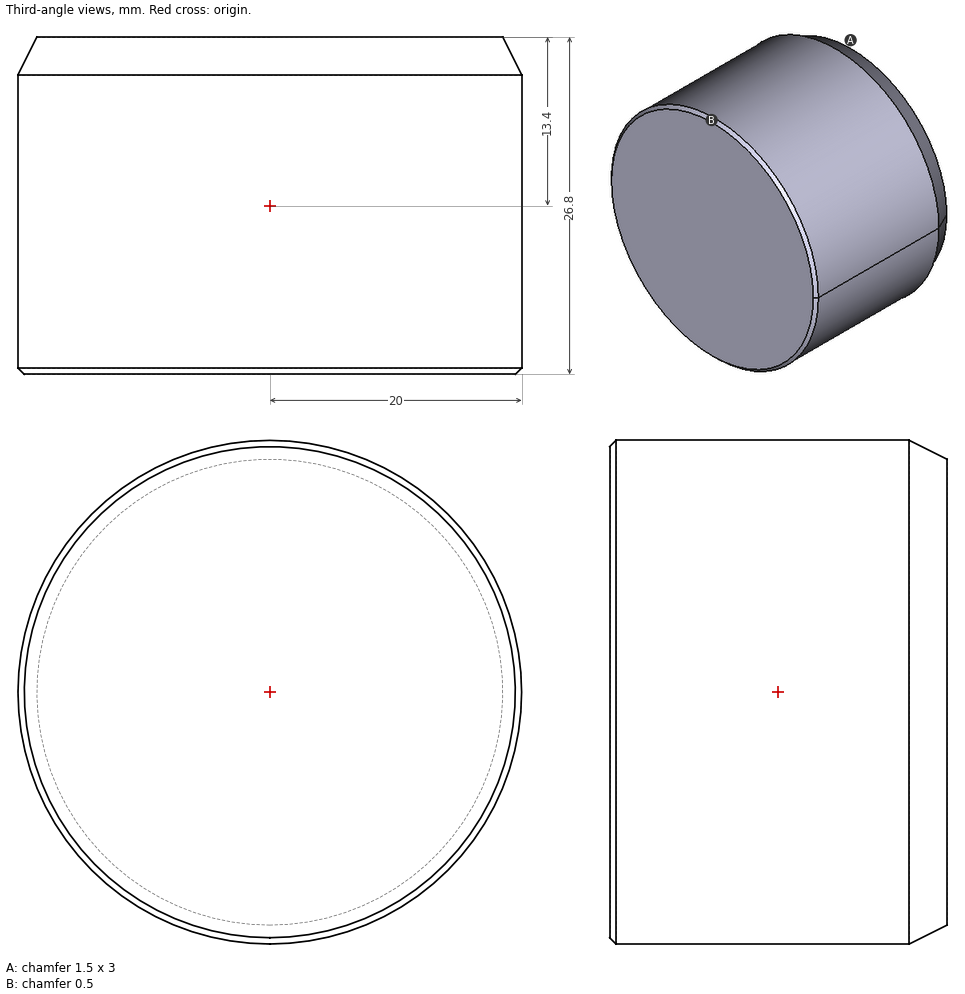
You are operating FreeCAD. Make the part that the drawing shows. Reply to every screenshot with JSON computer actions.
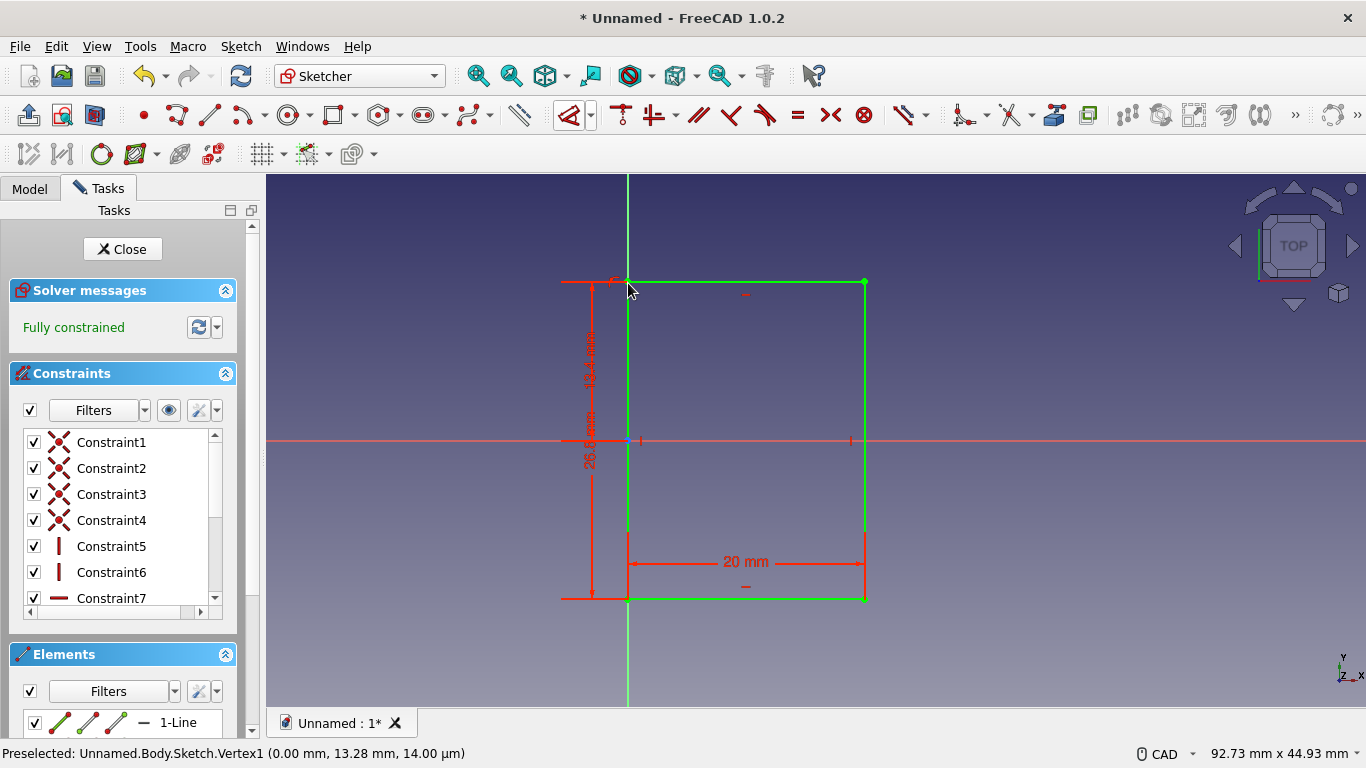
{"action": "left_click", "coordinate": [123, 249]}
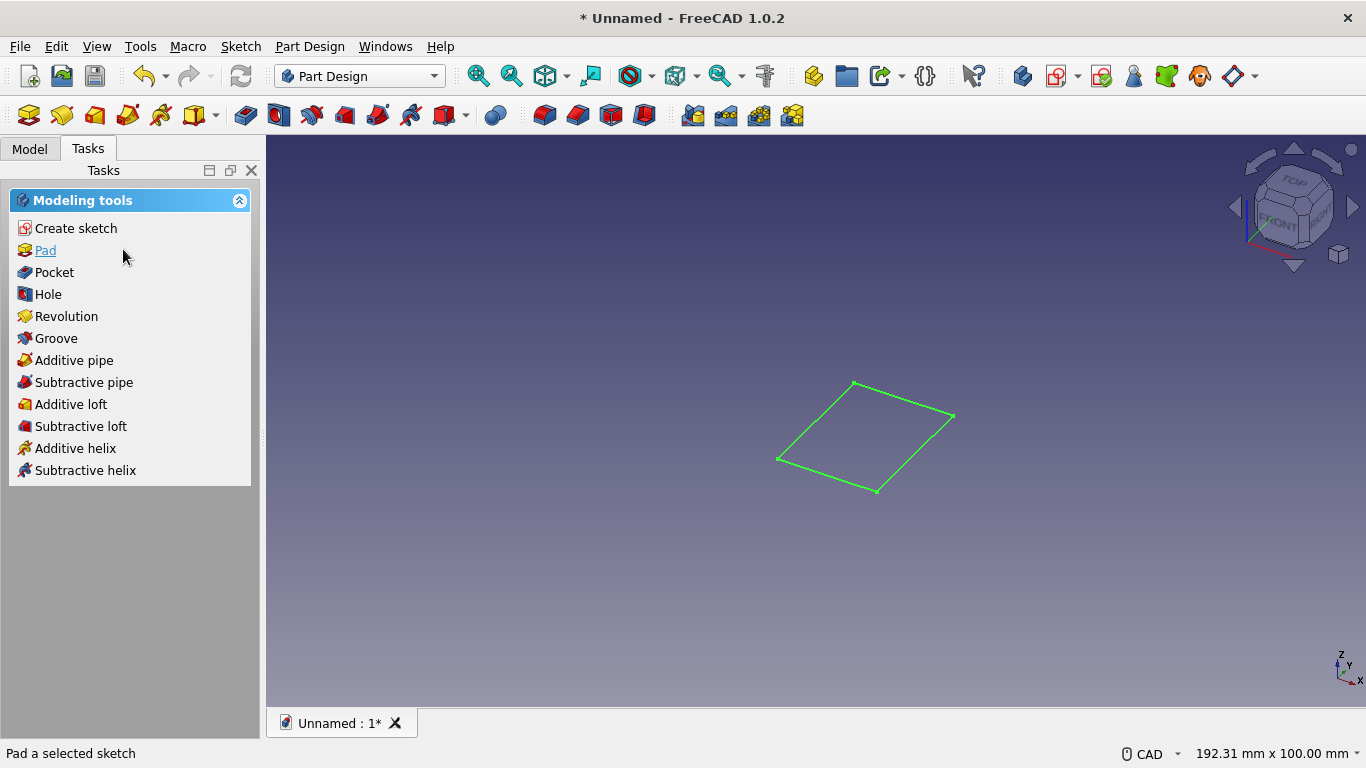
{"action": "left_click", "coordinate": [62, 116]}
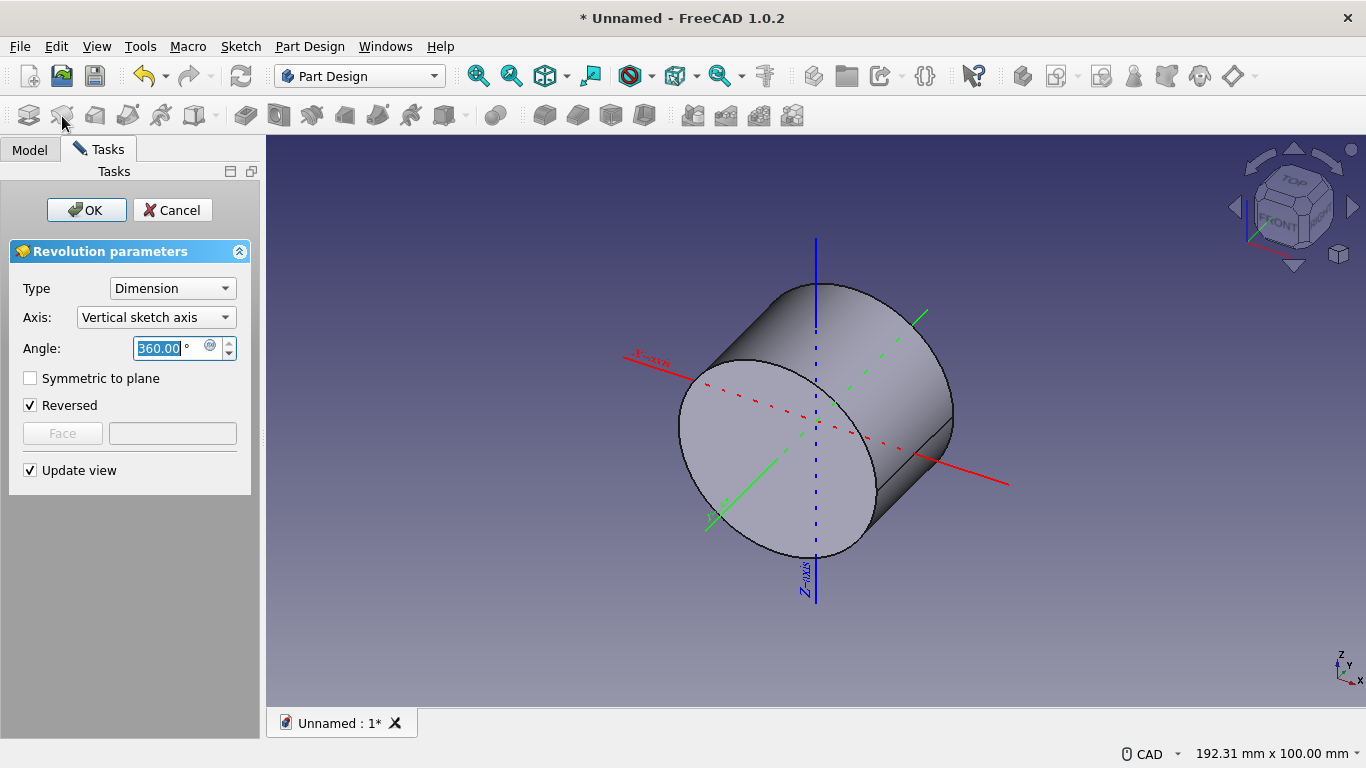
{"action": "left_click", "coordinate": [87, 210]}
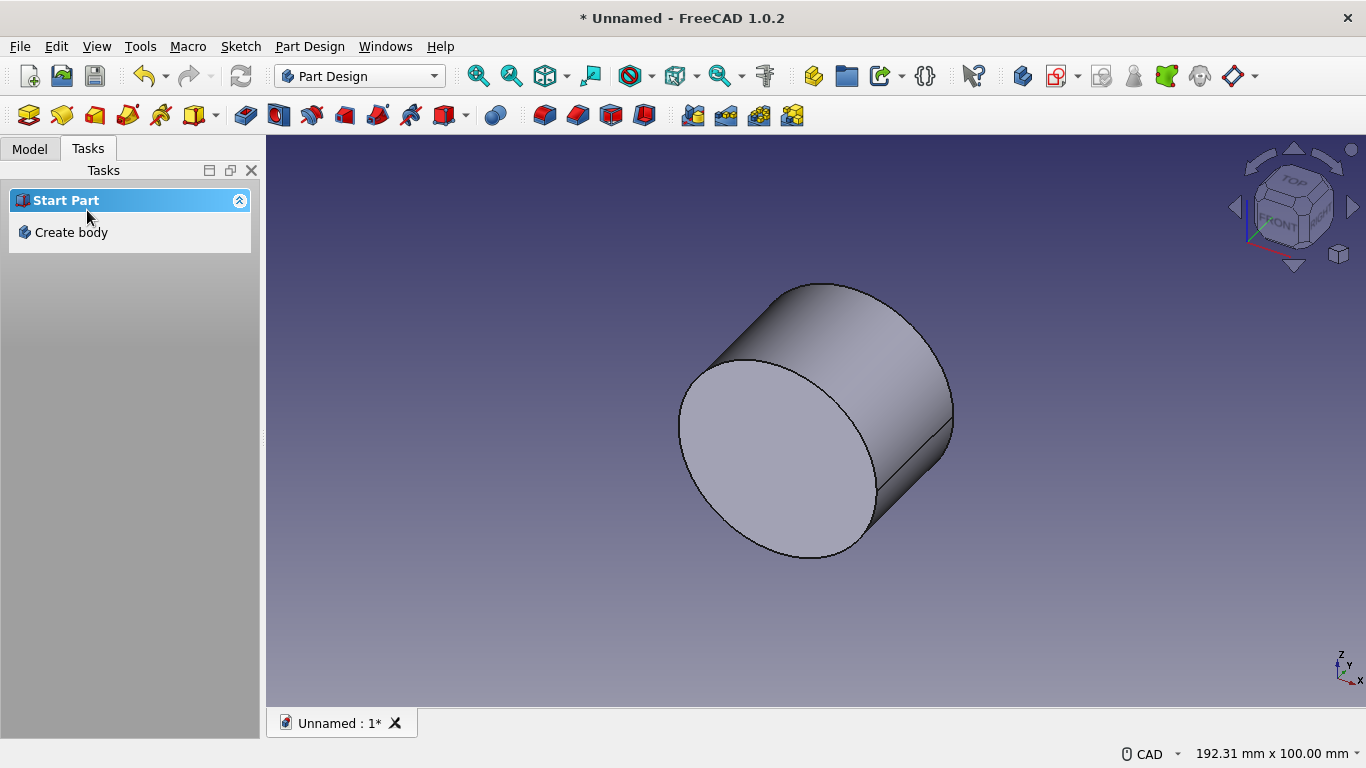
{"action": "key", "text": "0"}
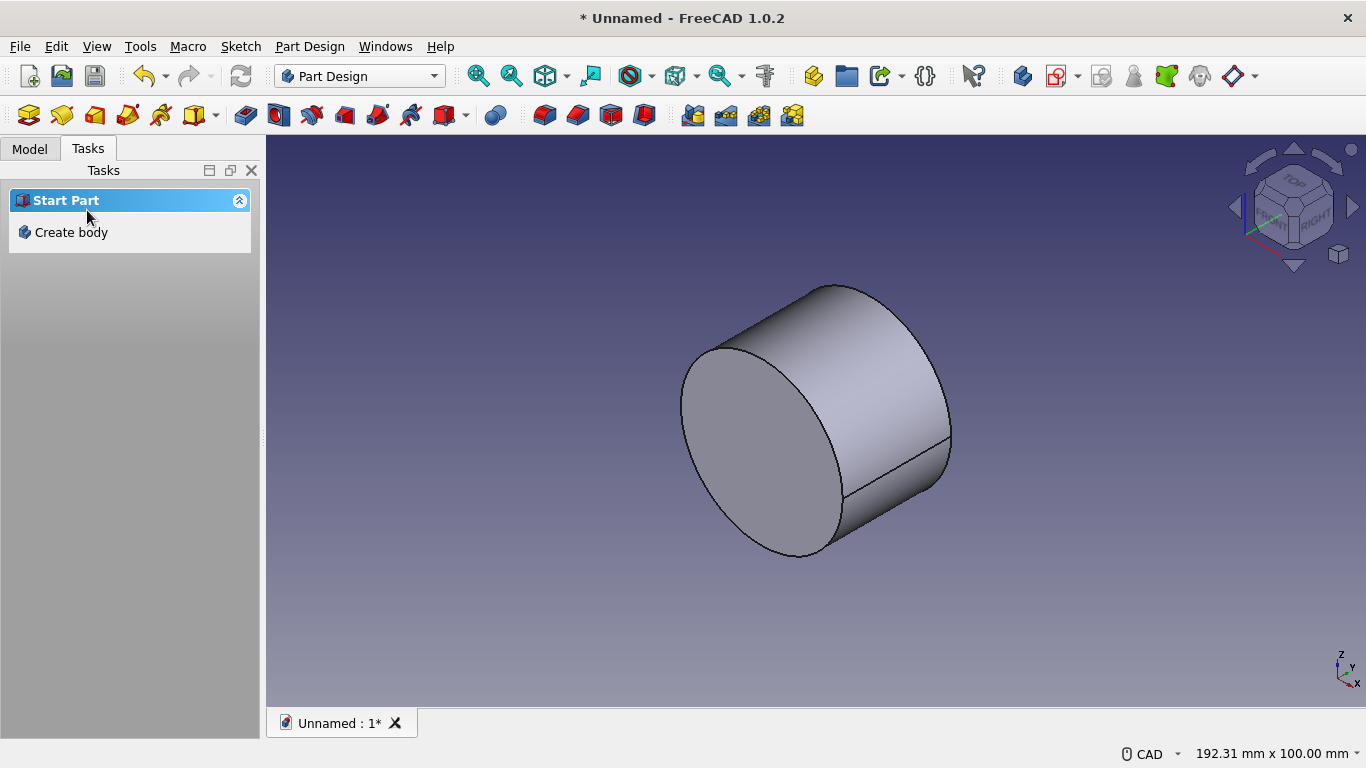
{"action": "key", "text": "2"}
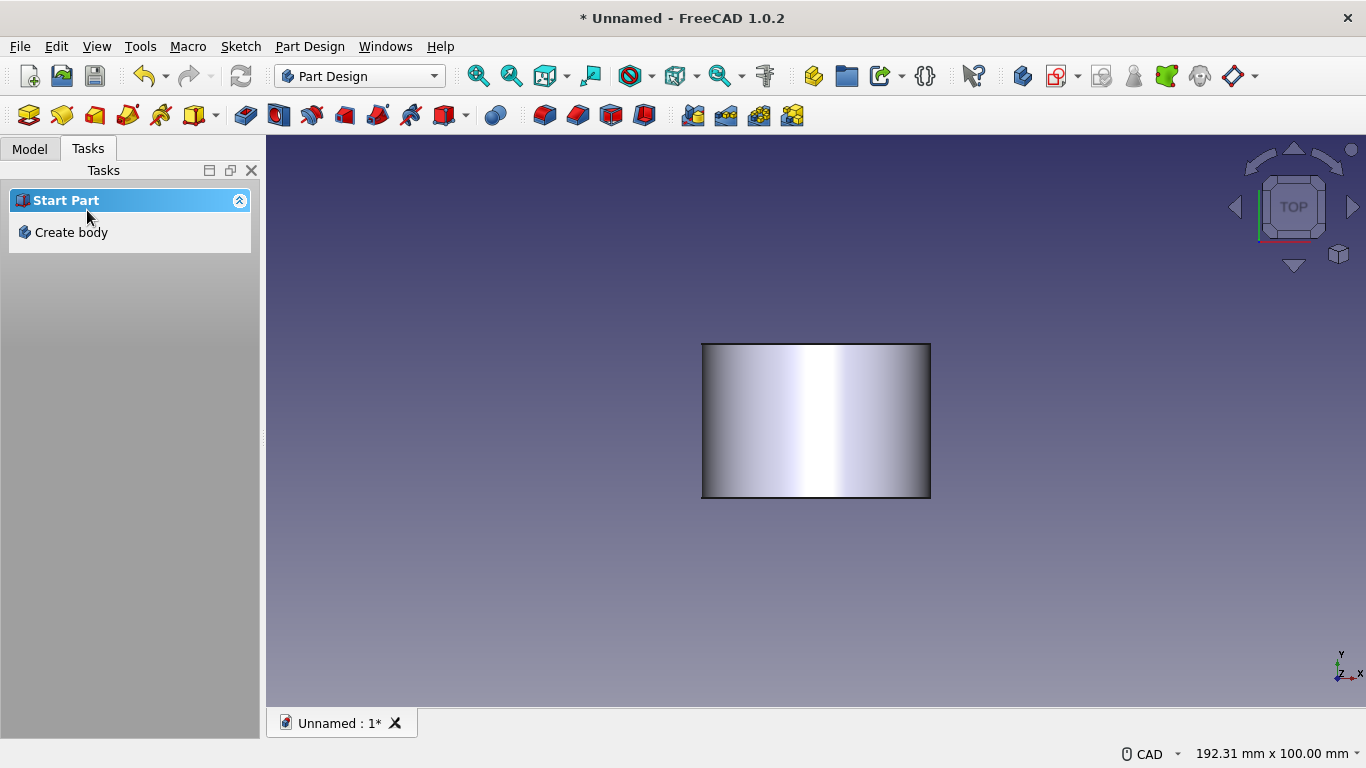
{"action": "key", "text": "v f"}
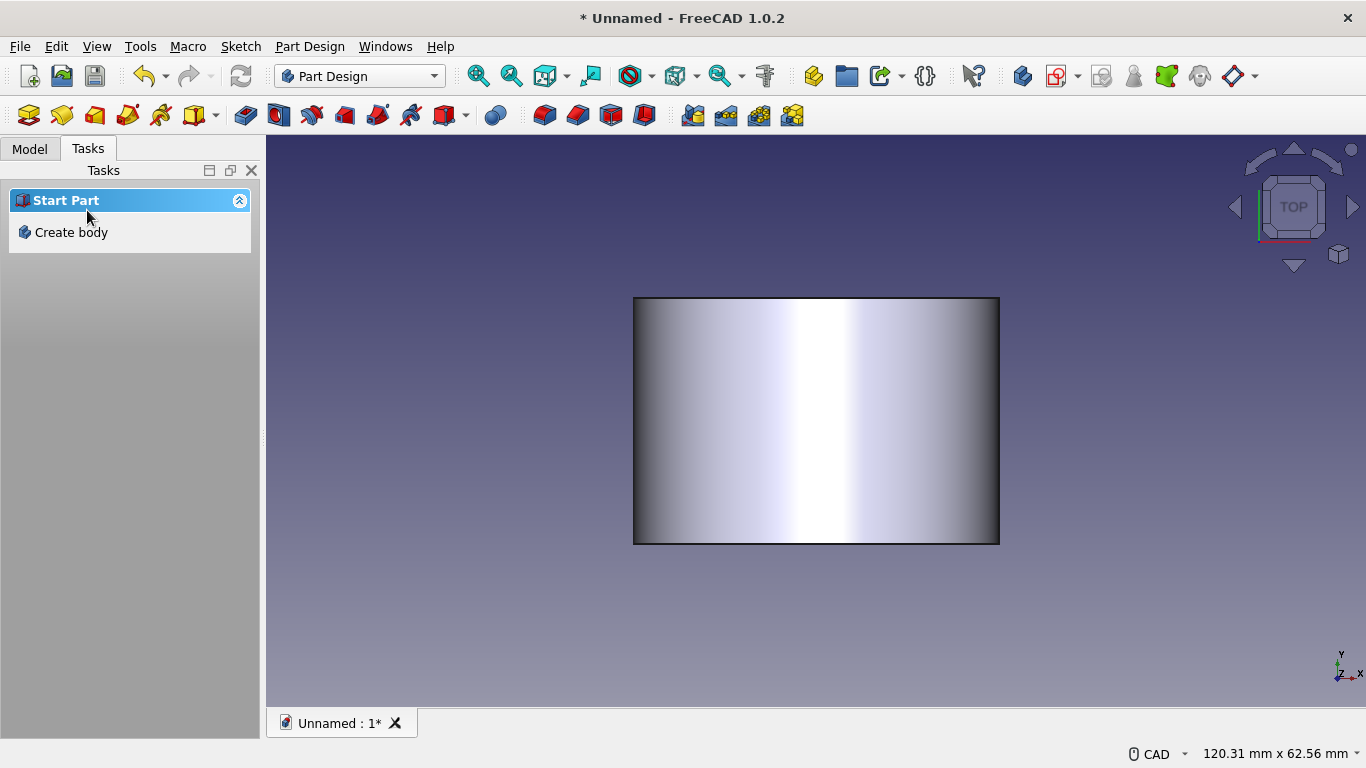
{"action": "left_click", "coordinate": [668, 297]}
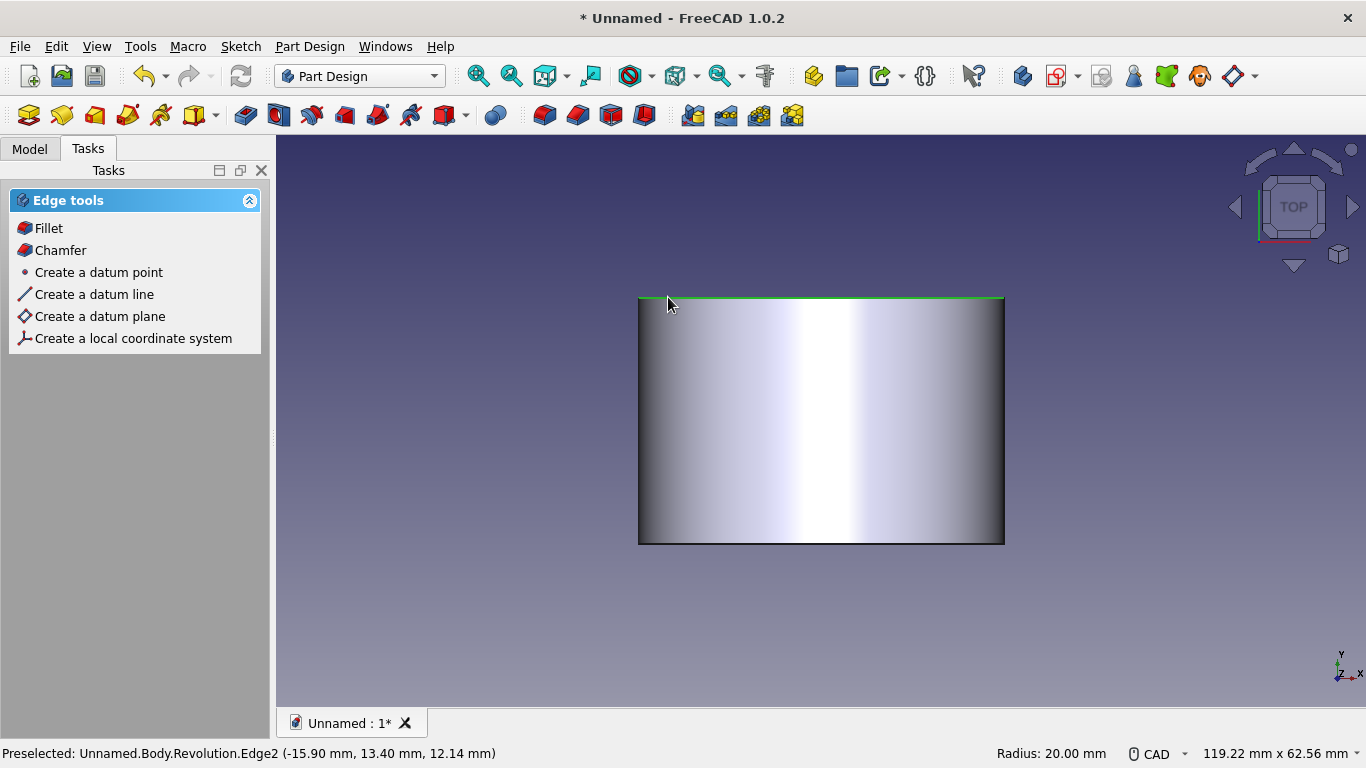
{"action": "left_click", "coordinate": [578, 116]}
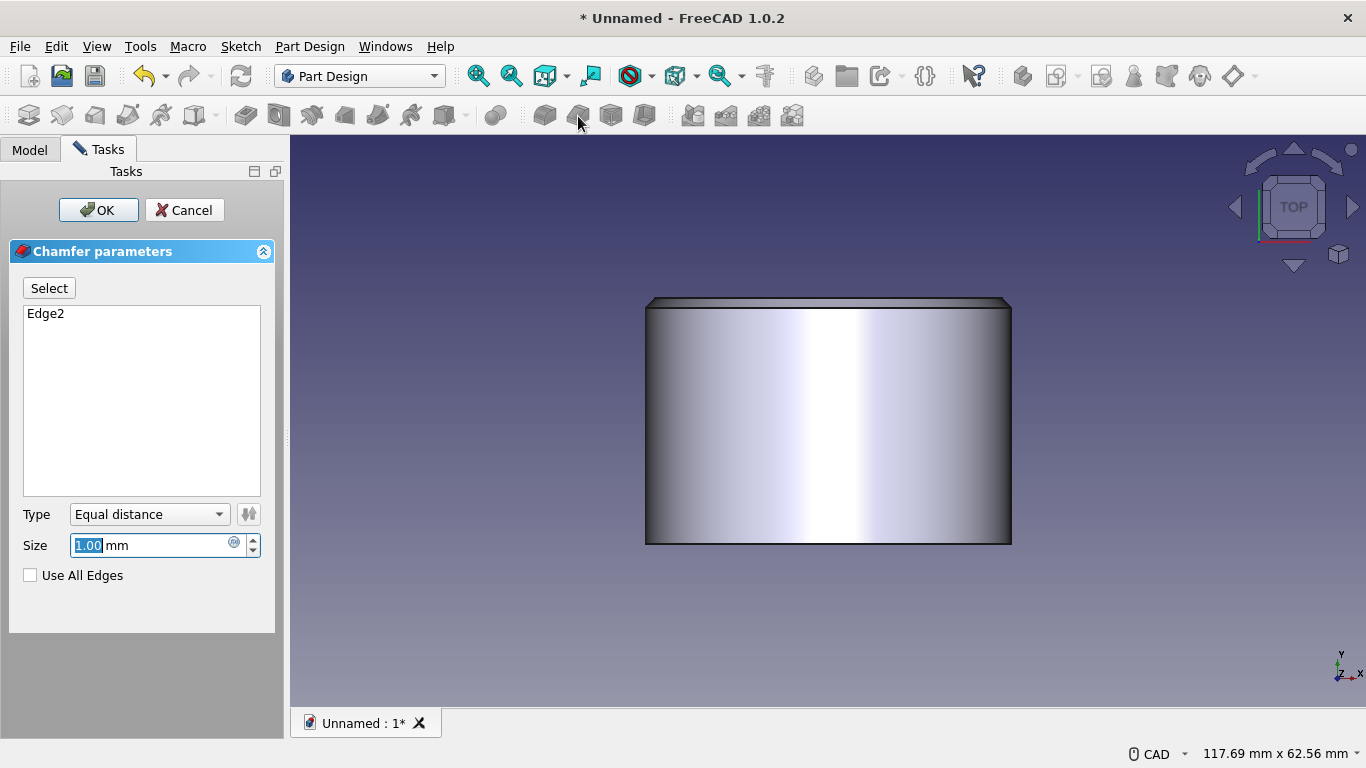
{"action": "type", "text": "1.5"}
{"action": "key", "text": "Tab"}